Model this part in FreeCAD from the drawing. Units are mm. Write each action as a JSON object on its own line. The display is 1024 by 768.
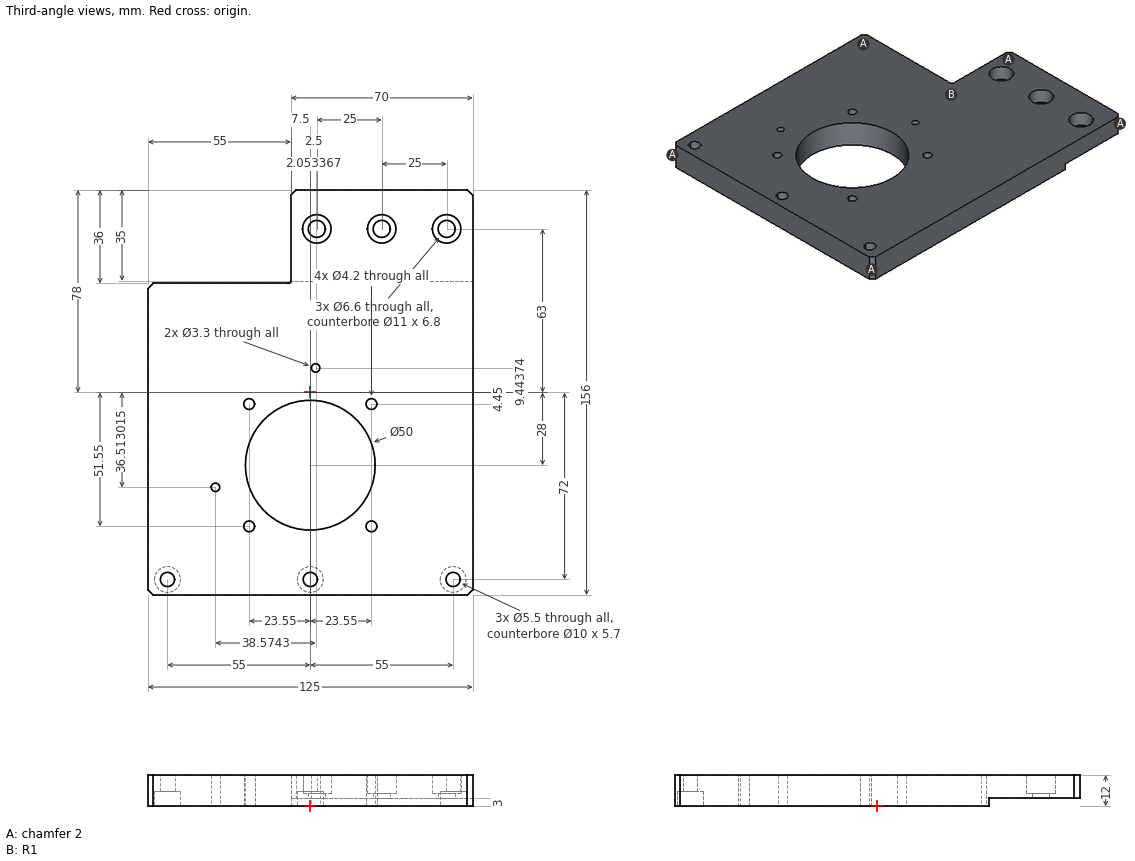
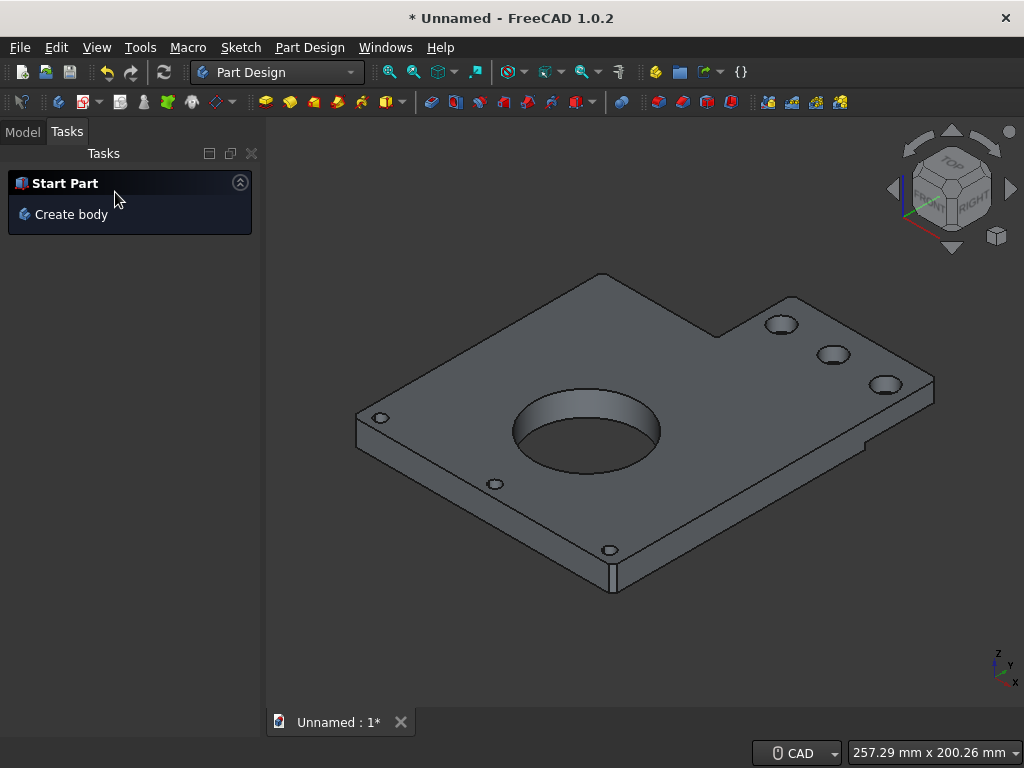
{"action": "left_click", "coordinate": [84, 102]}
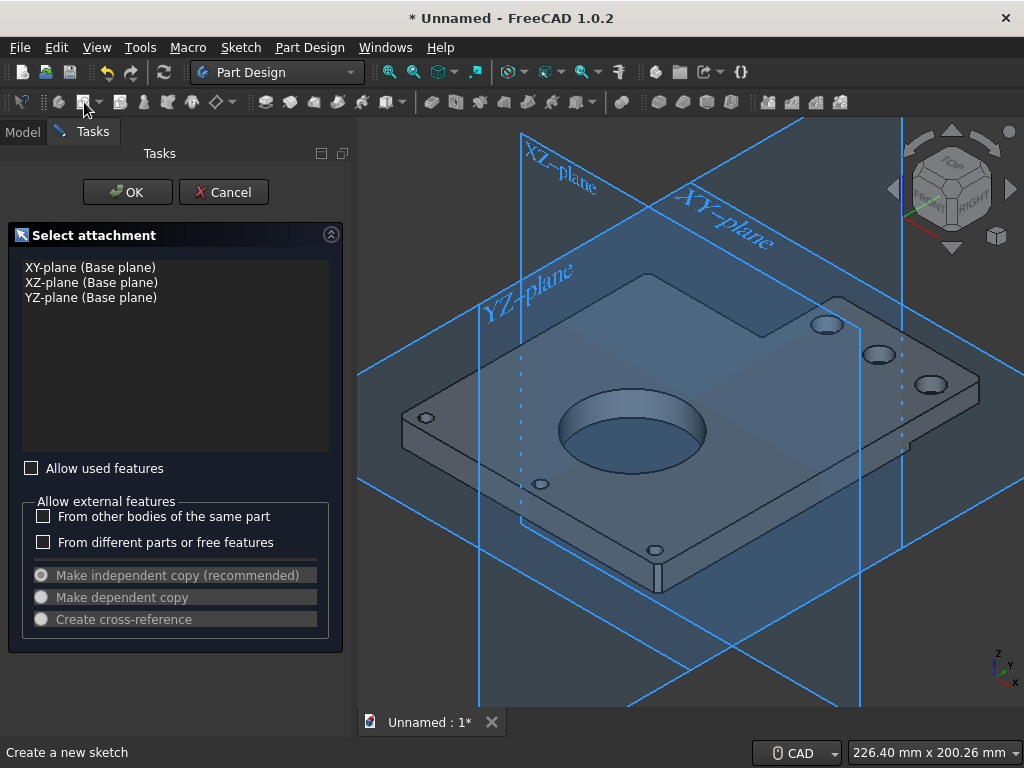
{"action": "left_click", "coordinate": [82, 268]}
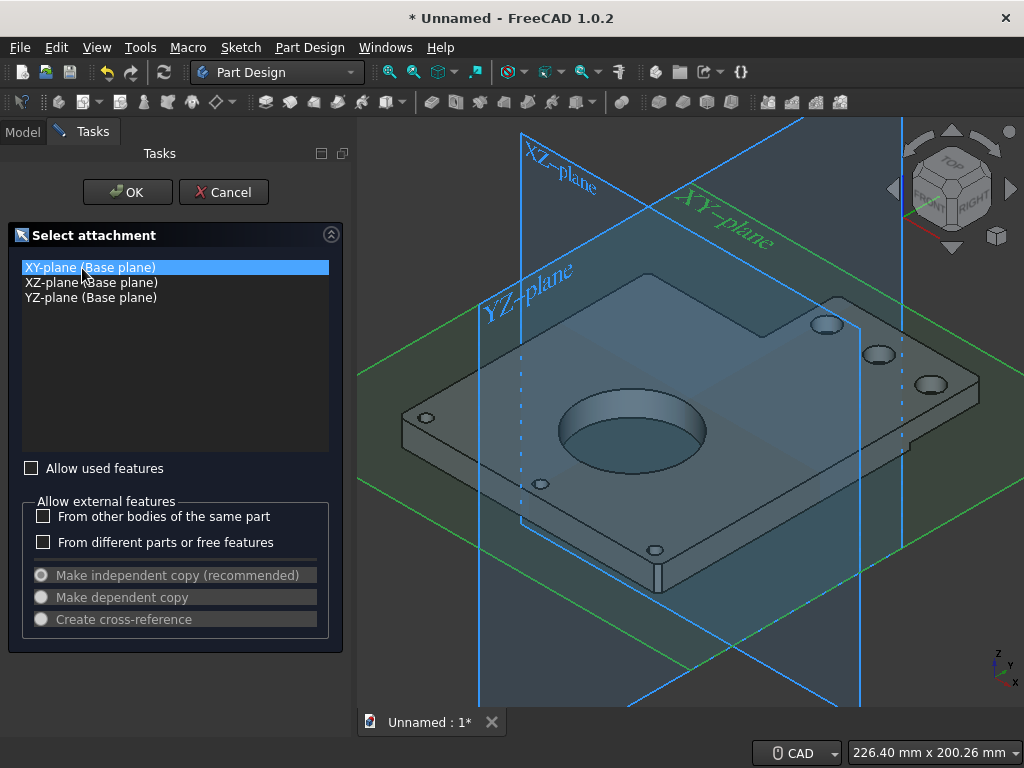
{"action": "left_click", "coordinate": [128, 192]}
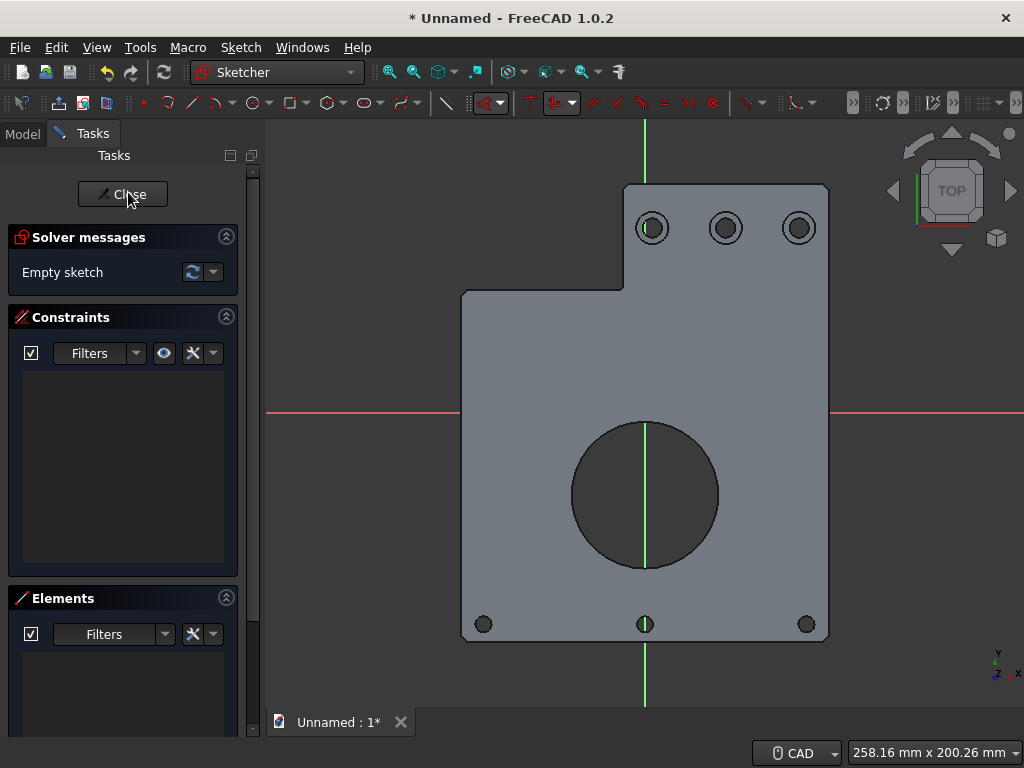
{"action": "left_click", "coordinate": [108, 104]}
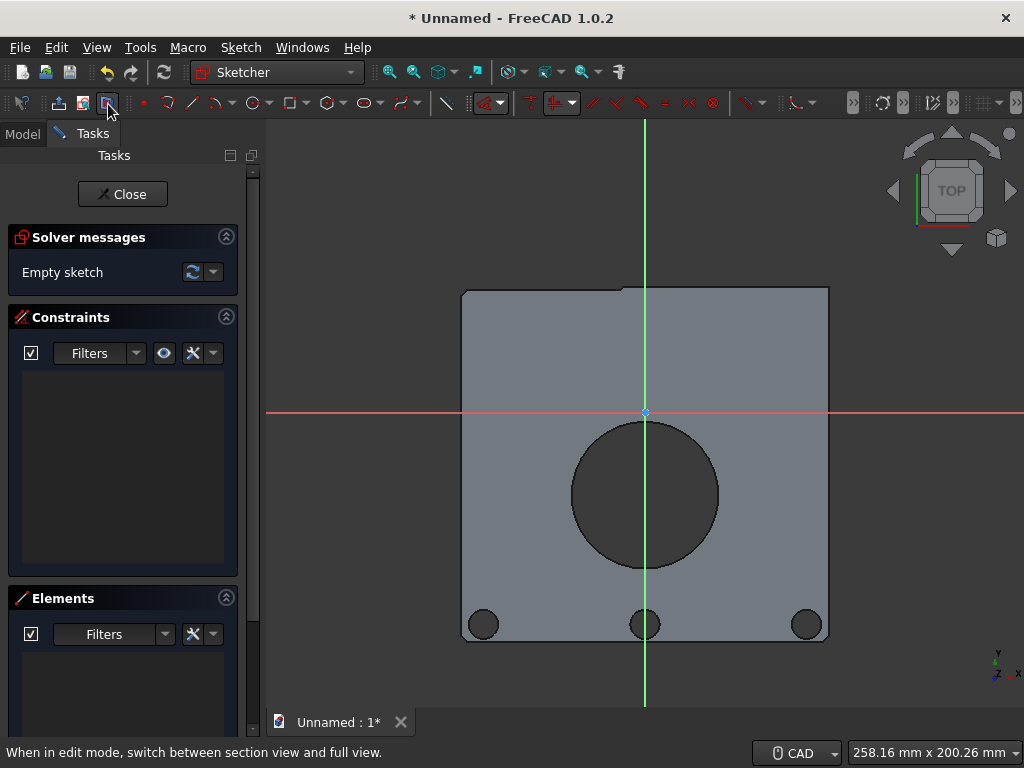
{"action": "scroll", "coordinate": [701, 556], "scroll_direction": "up", "scroll_amount": 4}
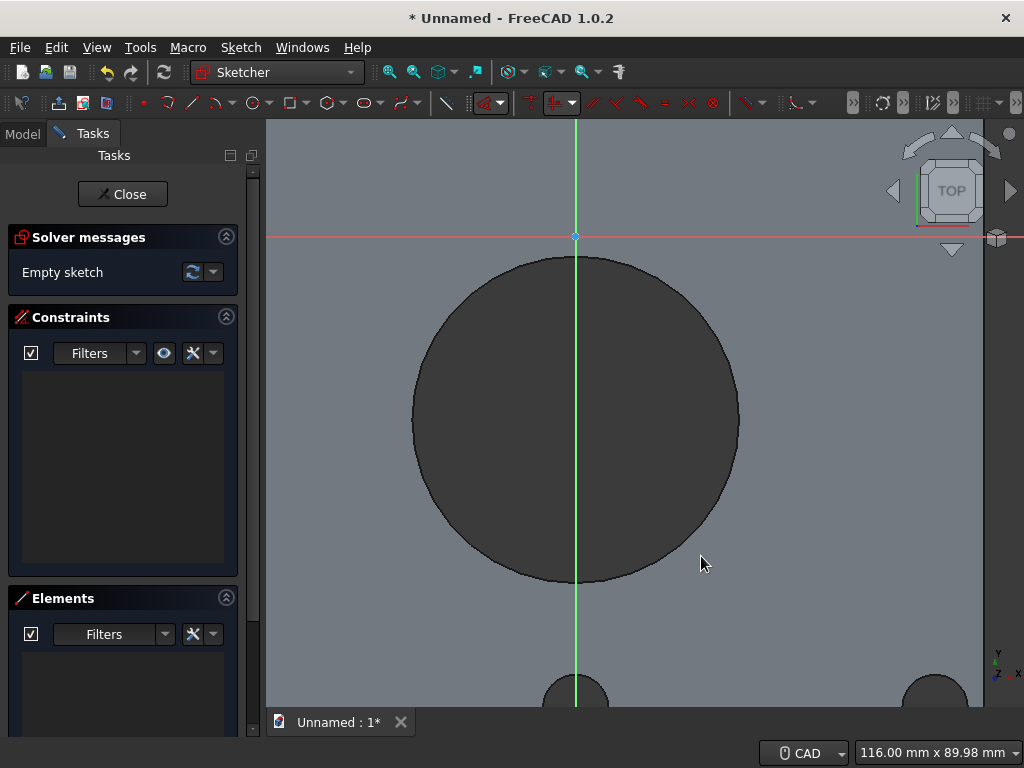
{"action": "left_click", "coordinate": [254, 104]}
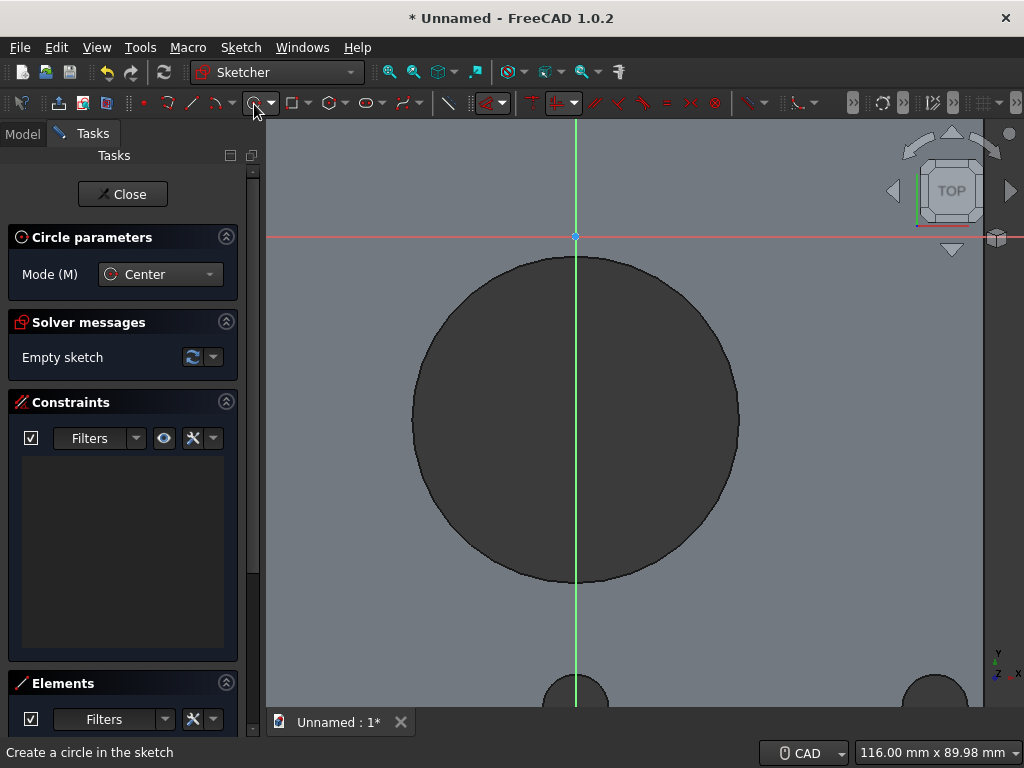
{"action": "scroll", "coordinate": [730, 266], "scroll_direction": "up", "scroll_amount": 3}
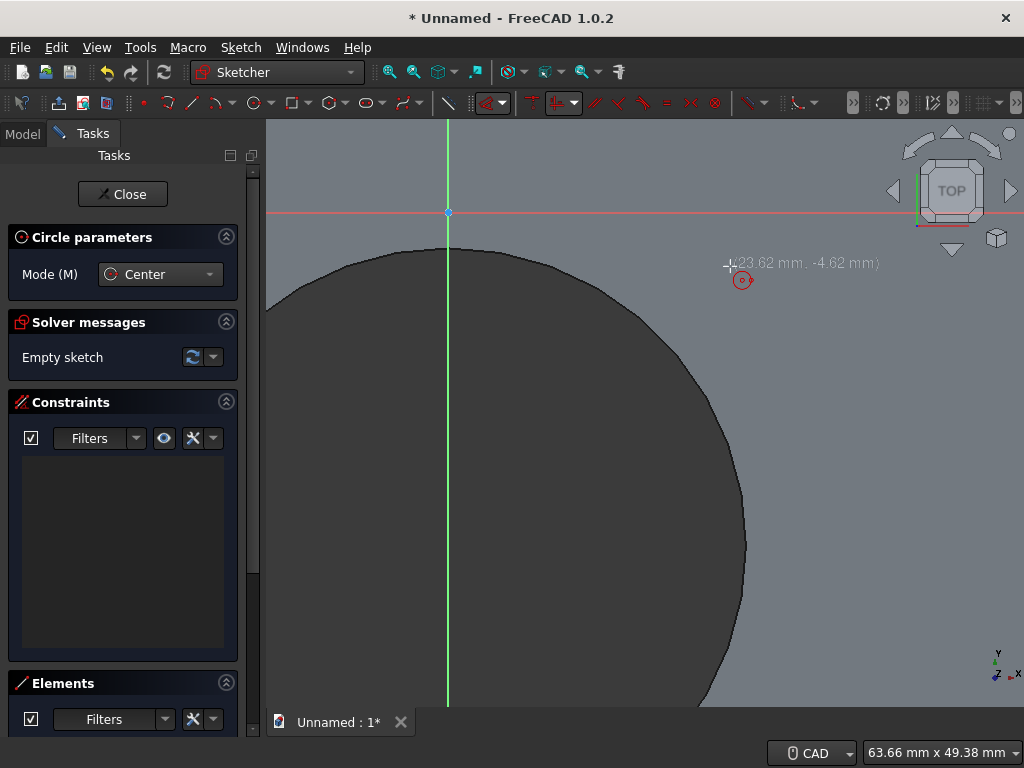
{"action": "left_click", "coordinate": [729, 266]}
{"action": "left_click", "coordinate": [746, 248]}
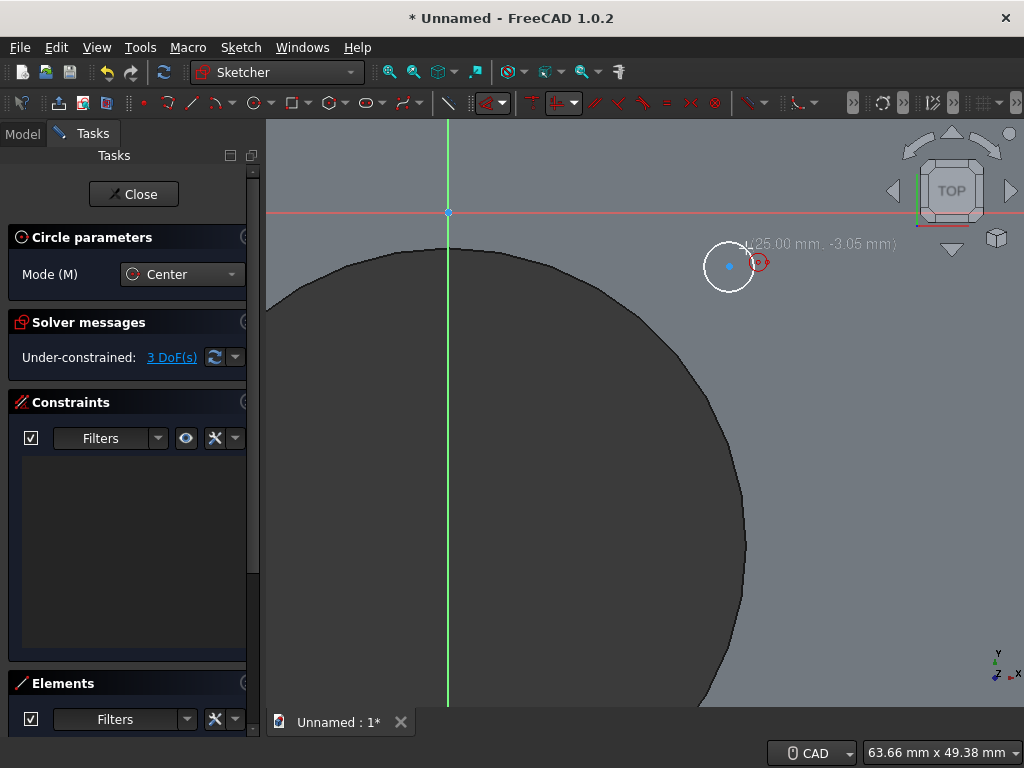
{"action": "scroll", "coordinate": [732, 268], "scroll_direction": "down", "scroll_amount": 3}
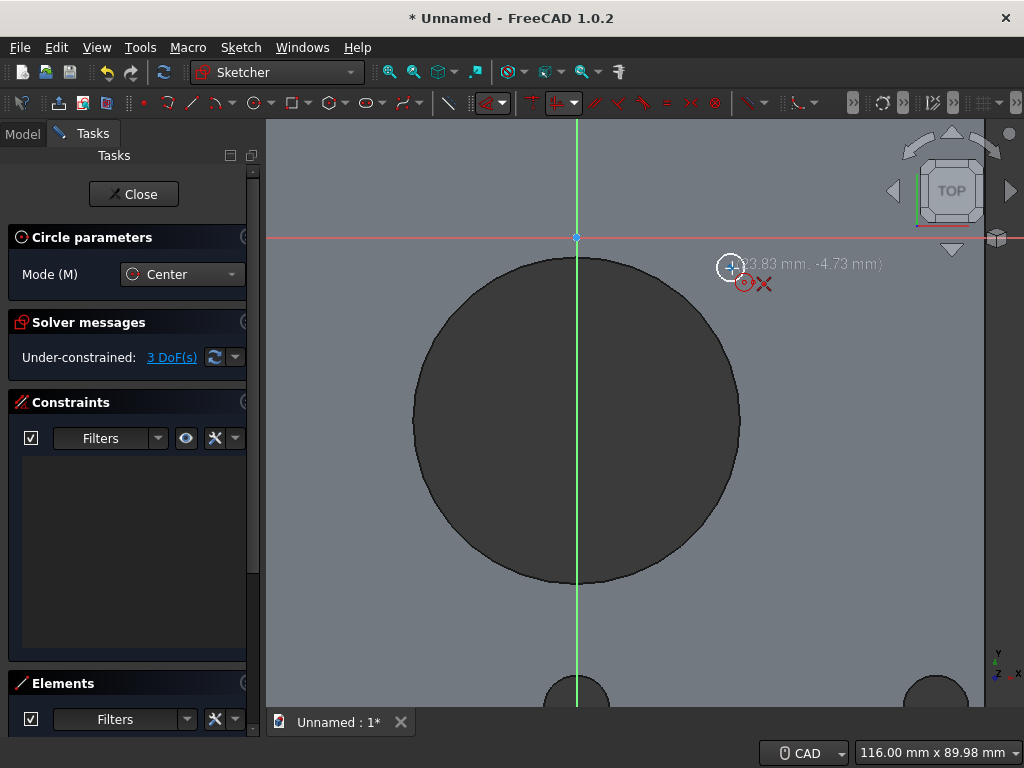
{"action": "scroll", "coordinate": [423, 267], "scroll_direction": "up", "scroll_amount": 3}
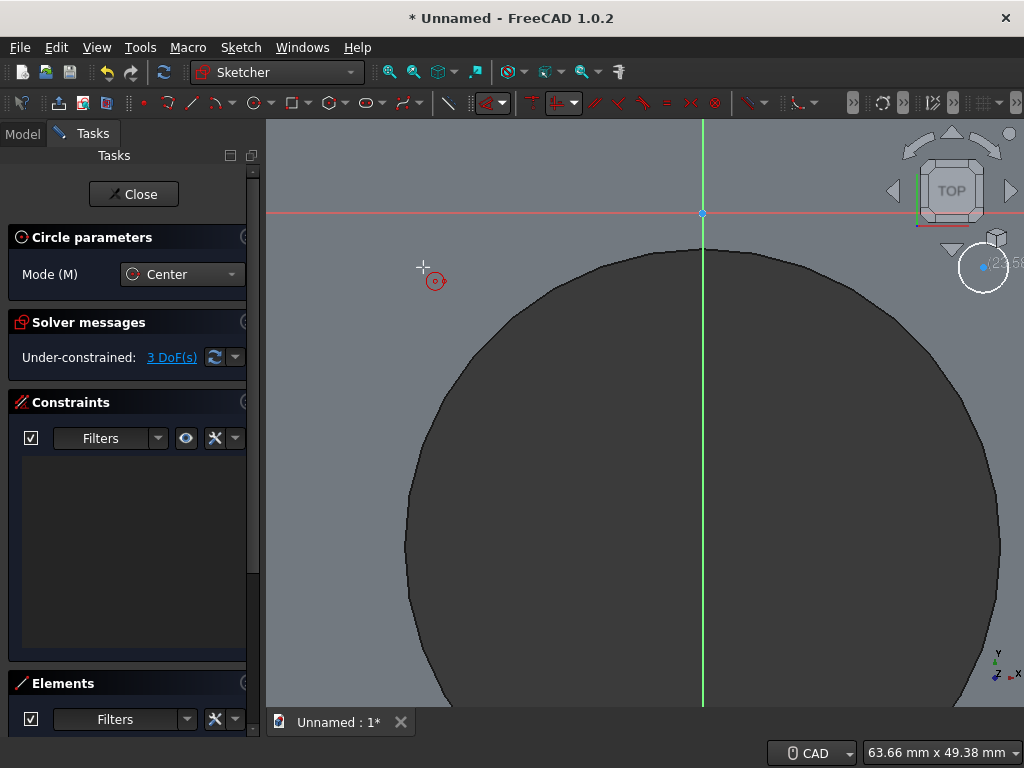
{"action": "left_click", "coordinate": [422, 266]}
{"action": "left_click", "coordinate": [440, 249]}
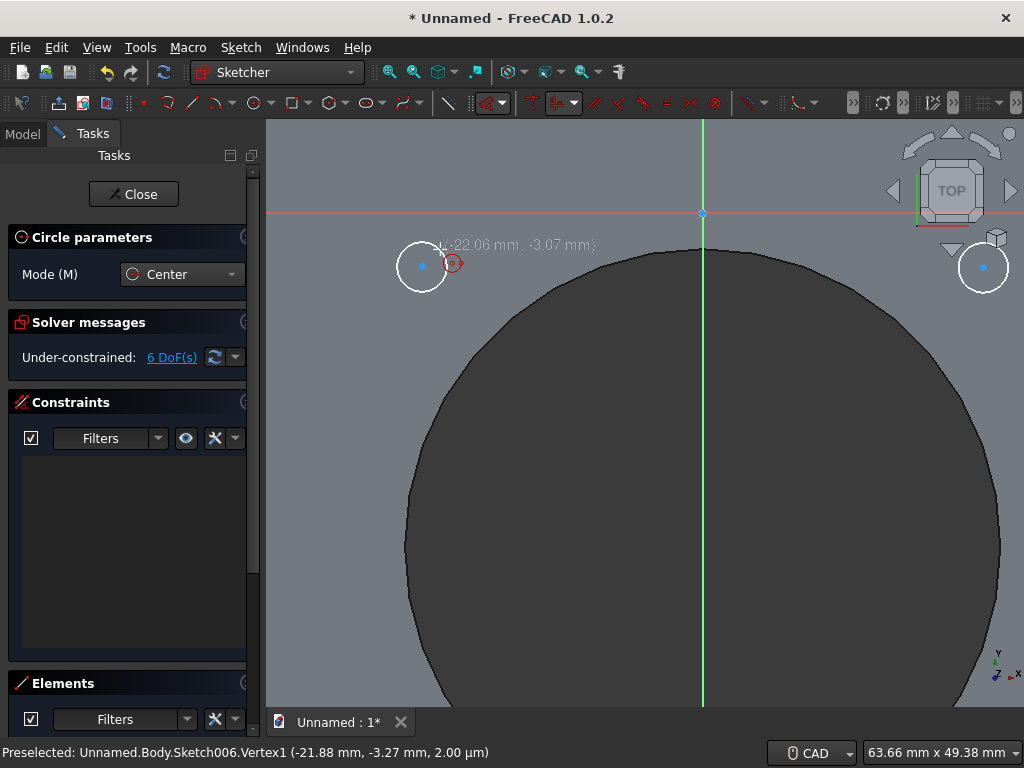
{"action": "scroll", "coordinate": [423, 267], "scroll_direction": "down", "scroll_amount": 3}